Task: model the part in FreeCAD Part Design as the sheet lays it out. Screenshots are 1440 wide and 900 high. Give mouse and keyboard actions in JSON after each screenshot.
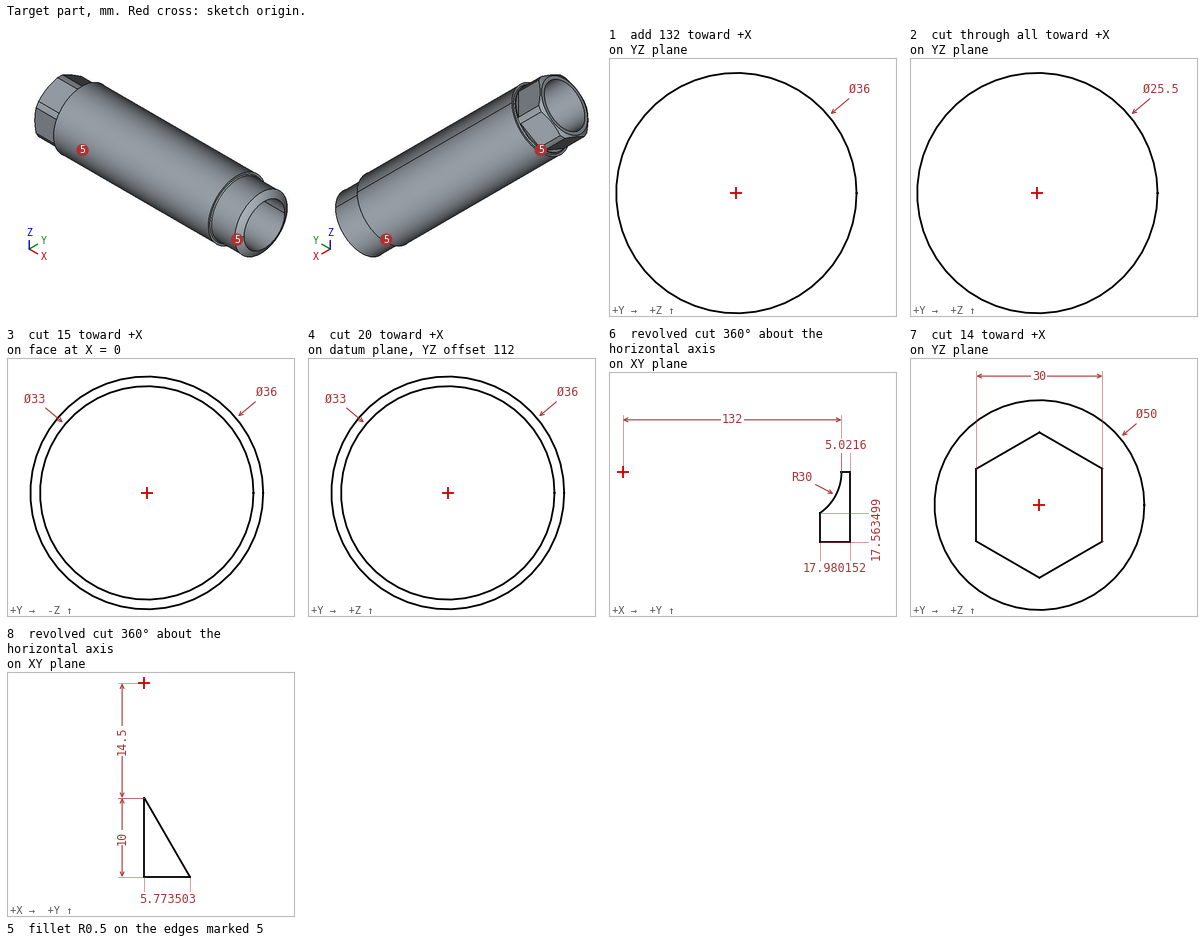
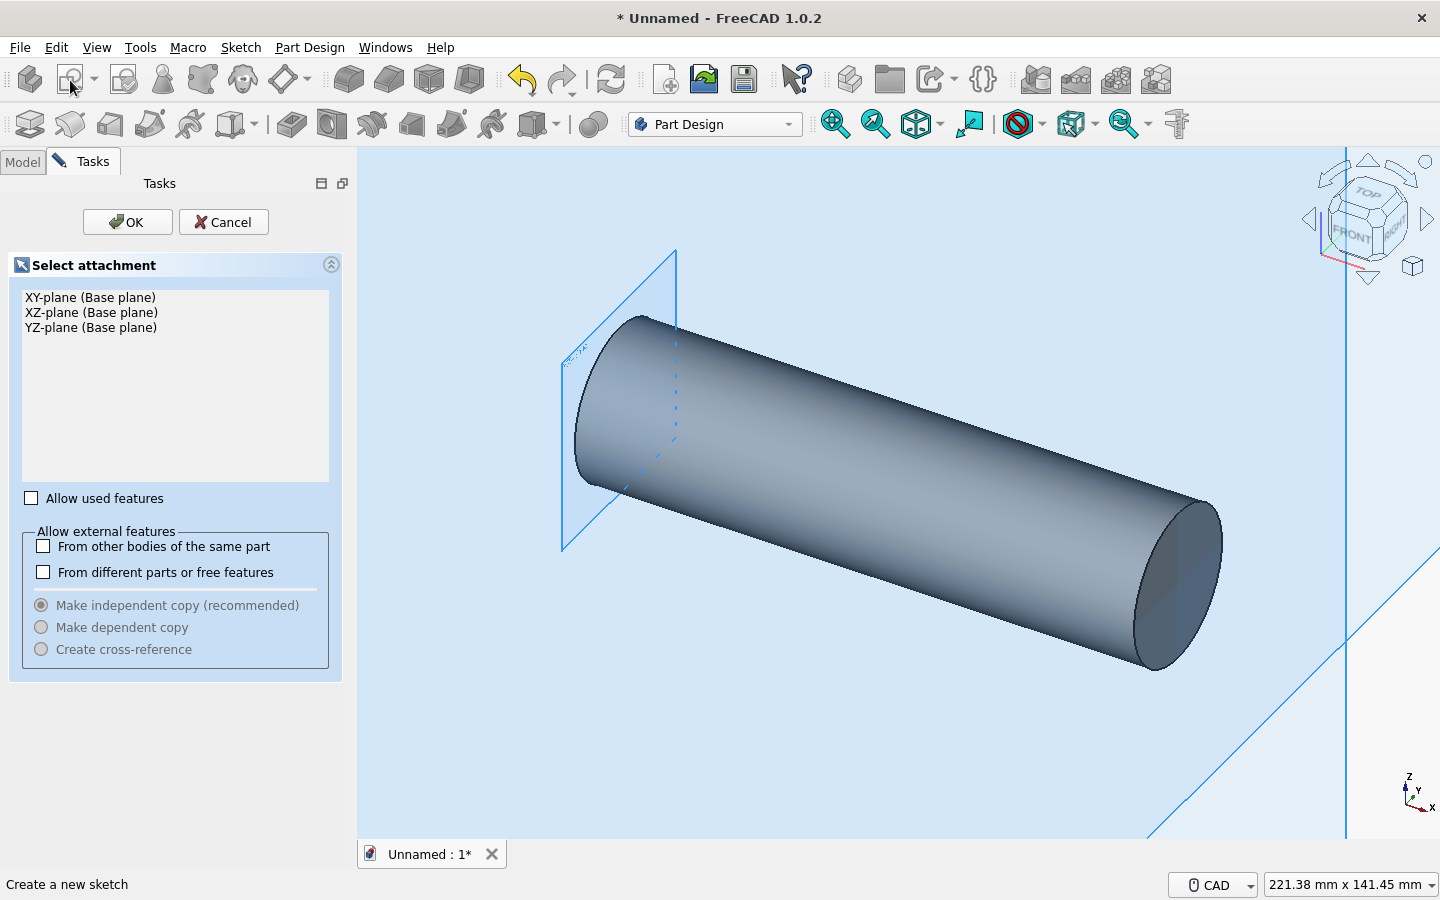
{"action": "left_click", "coordinate": [82, 328]}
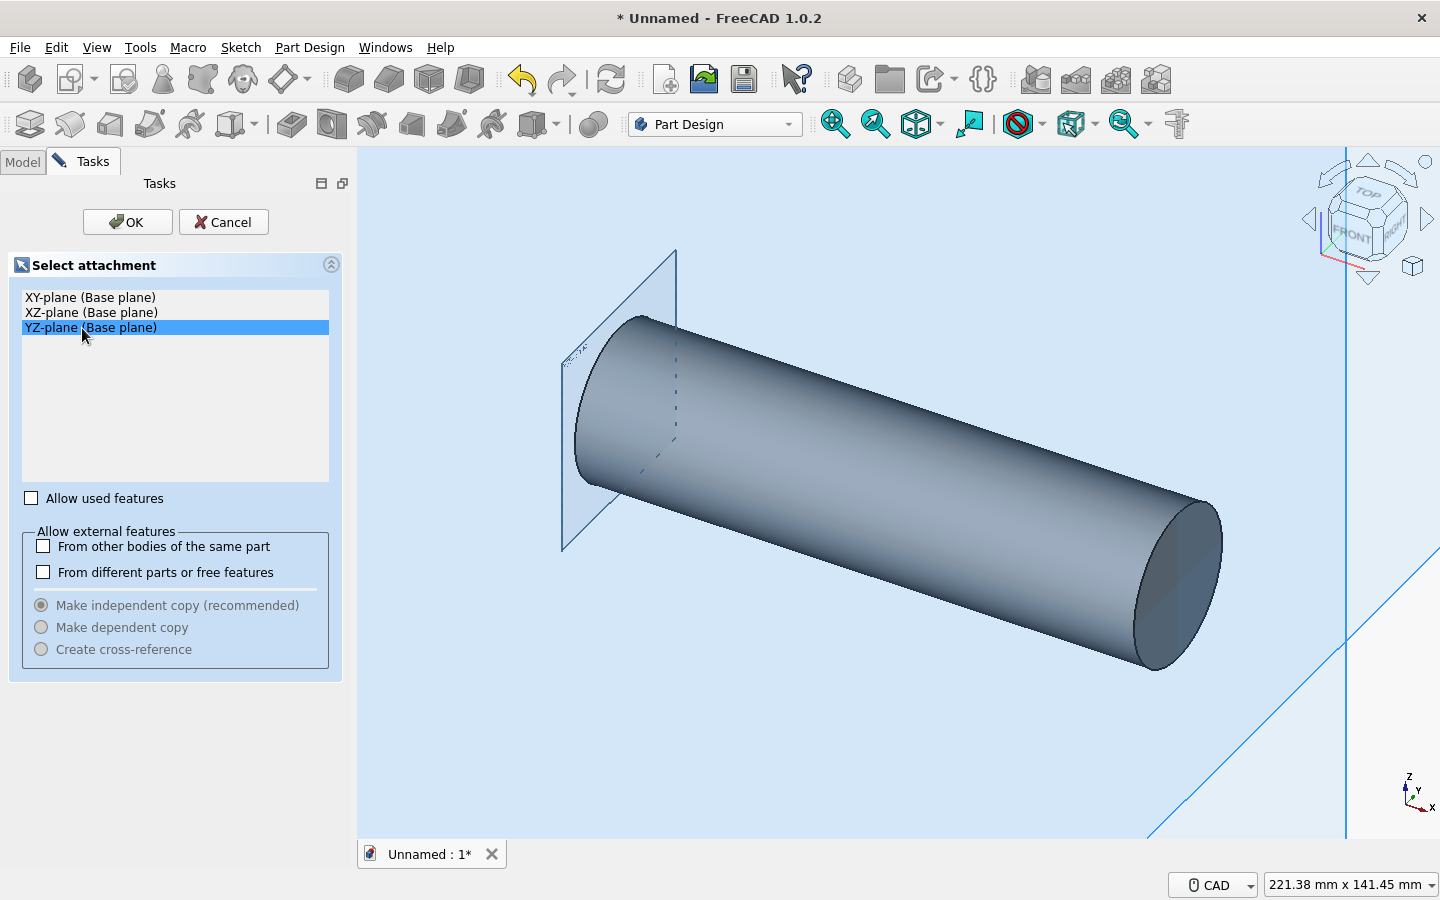
{"action": "left_click", "coordinate": [128, 222]}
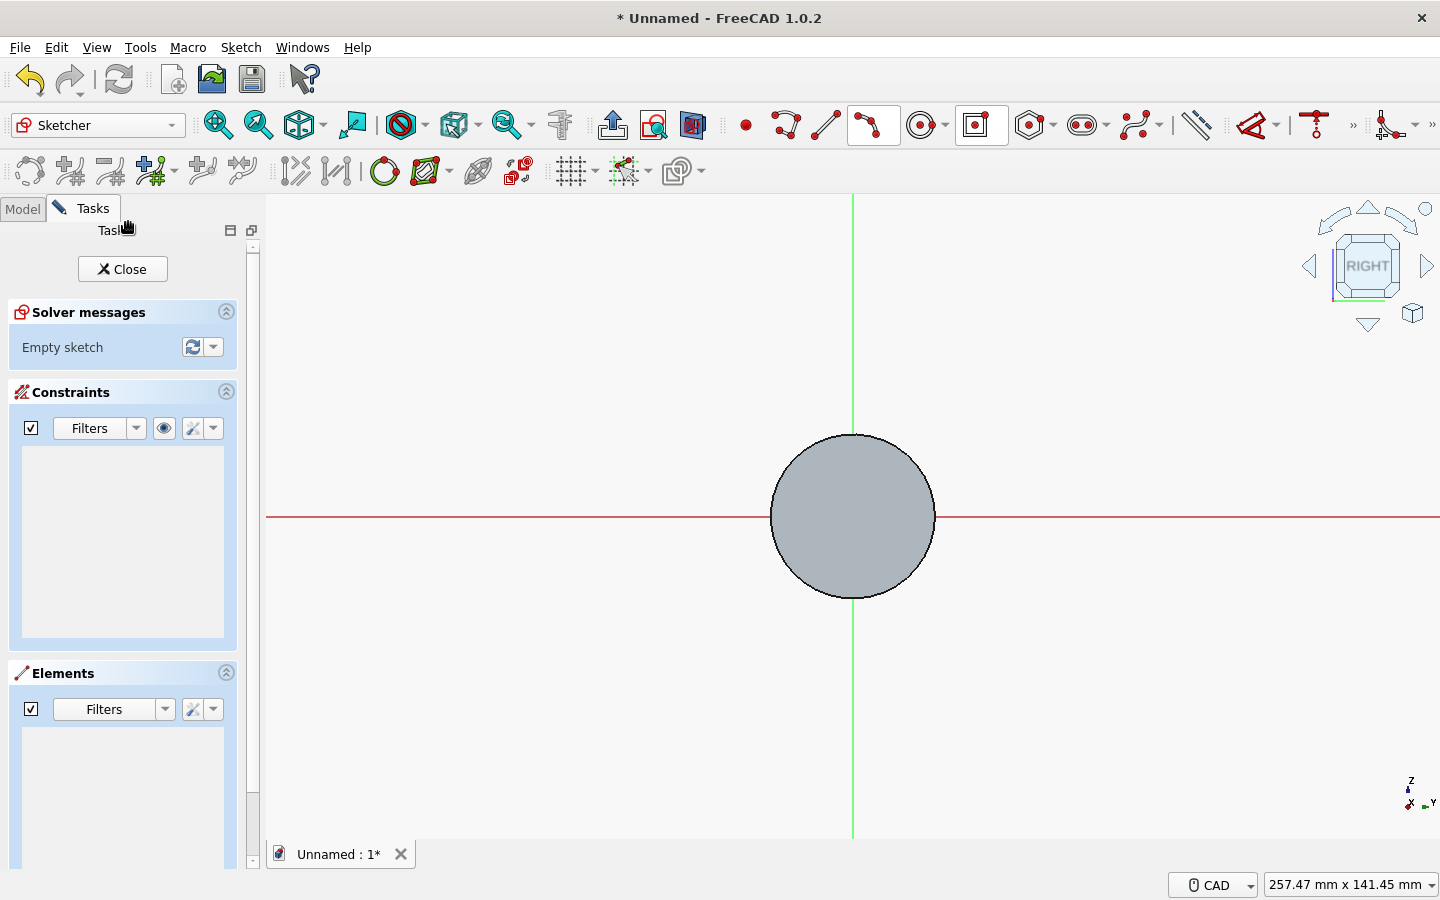
{"action": "key", "text": "q s"}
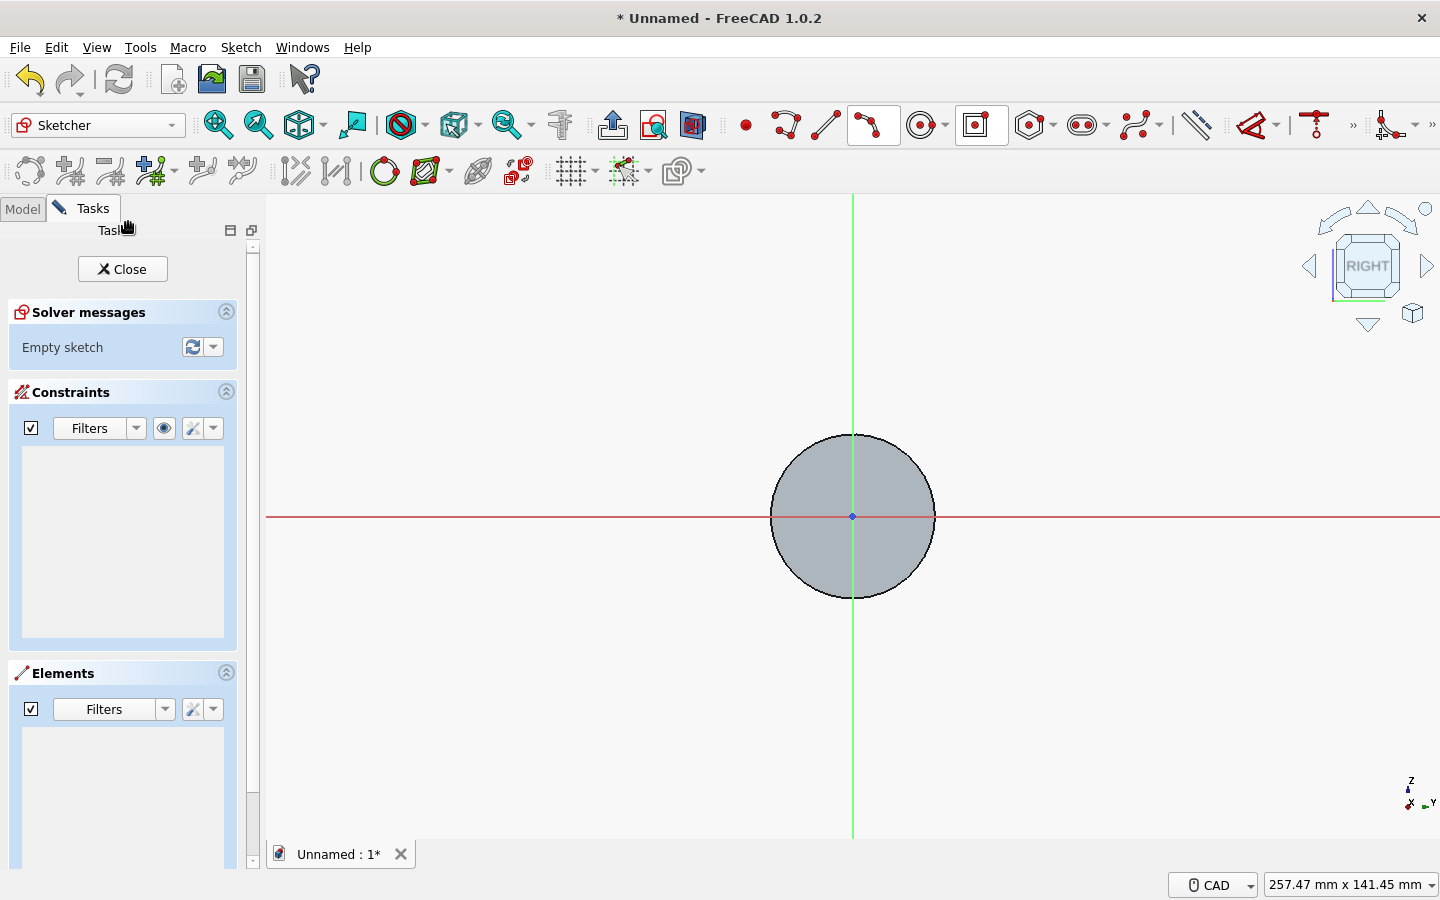
{"action": "scroll", "coordinate": [882, 516], "scroll_direction": "up", "scroll_amount": 6}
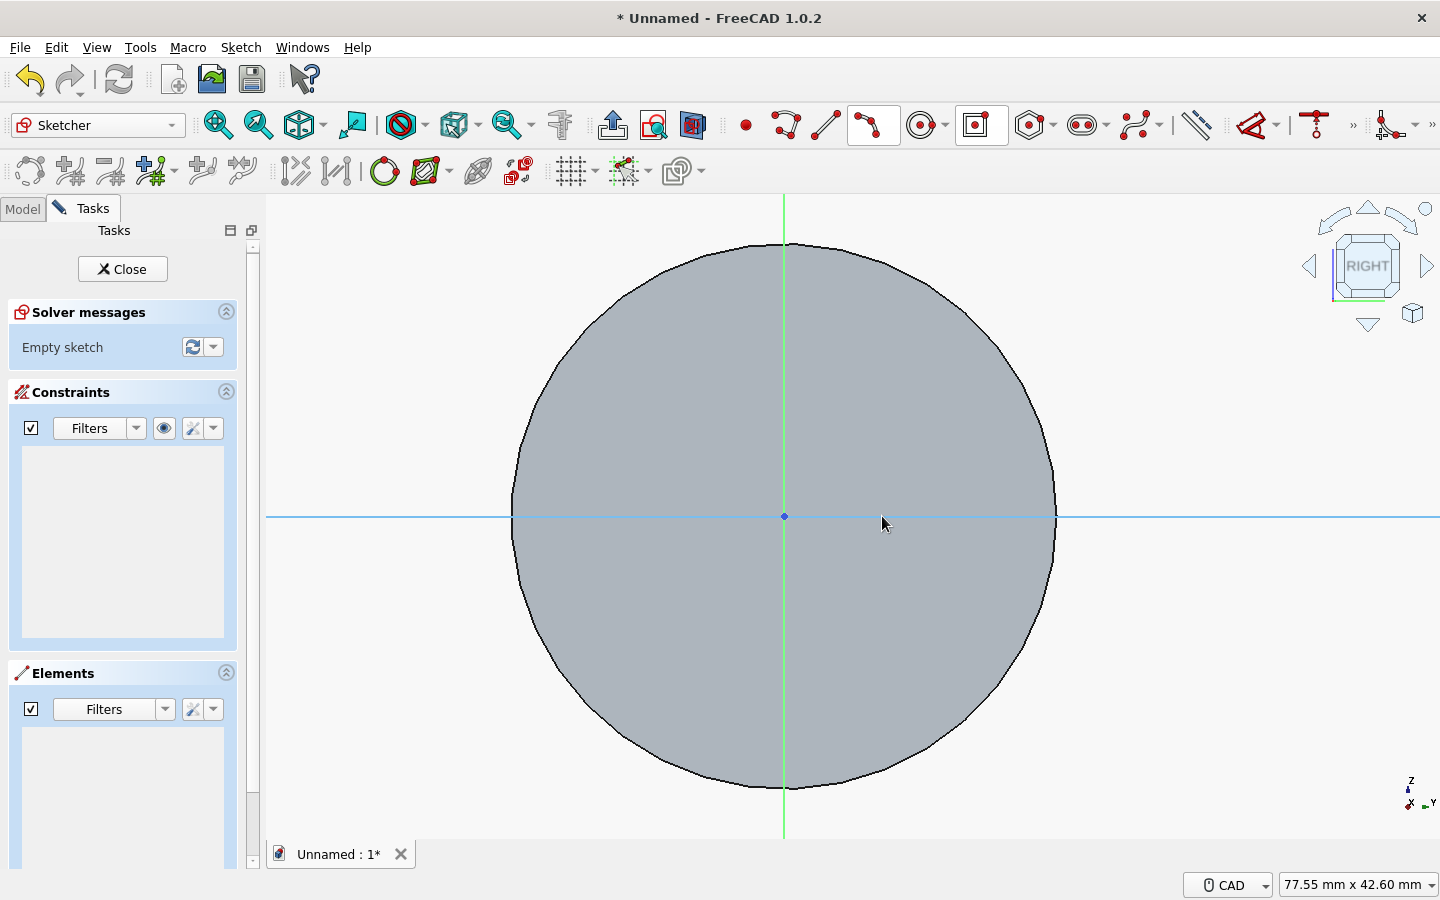
{"action": "left_click", "coordinate": [922, 126]}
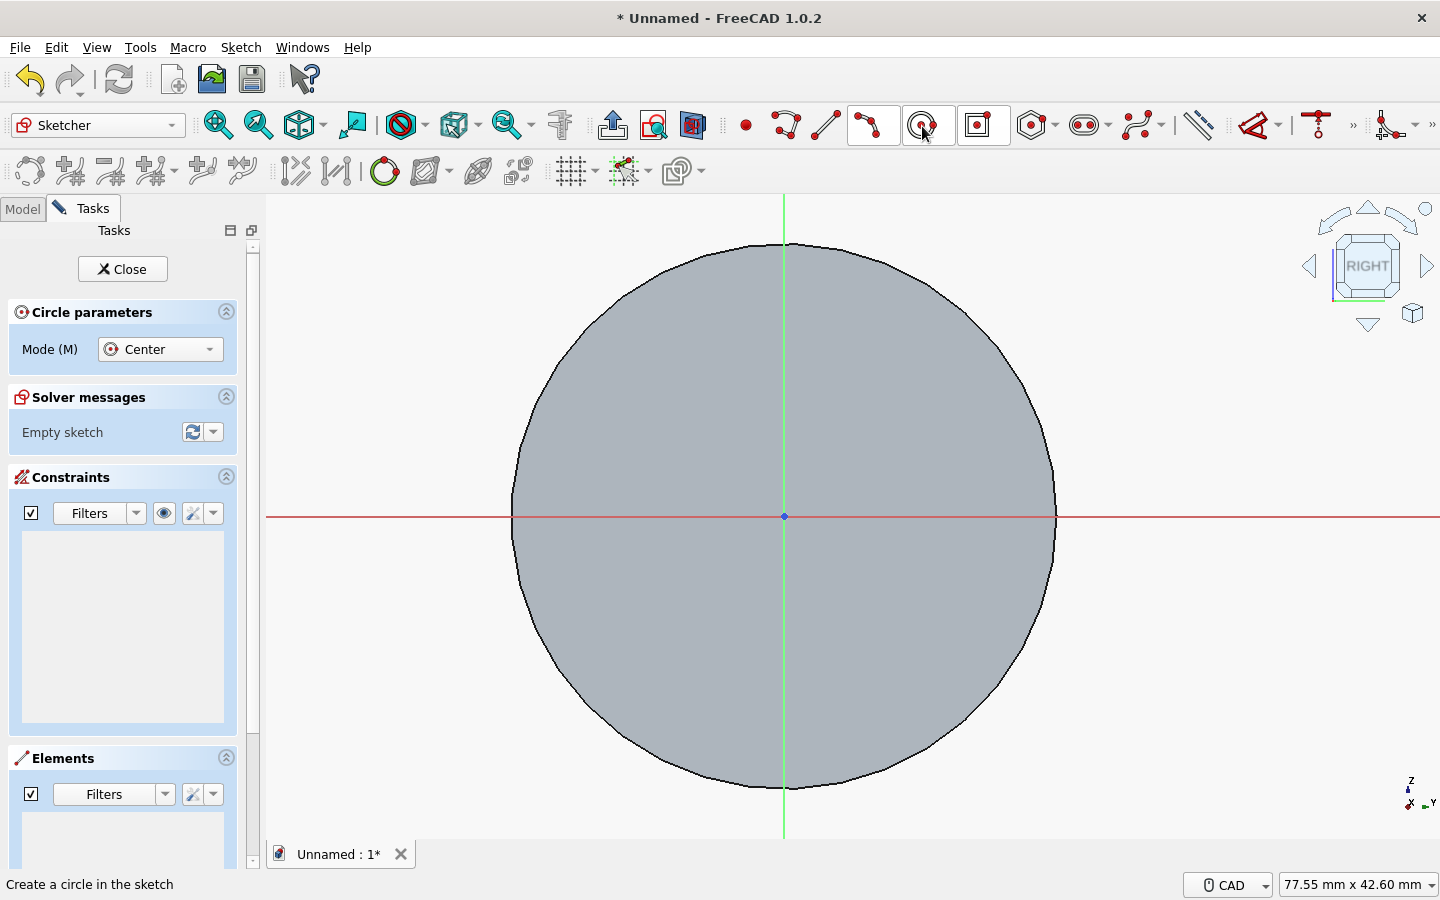
{"action": "left_click", "coordinate": [784, 516]}
{"action": "mouse_move", "coordinate": [920, 380]}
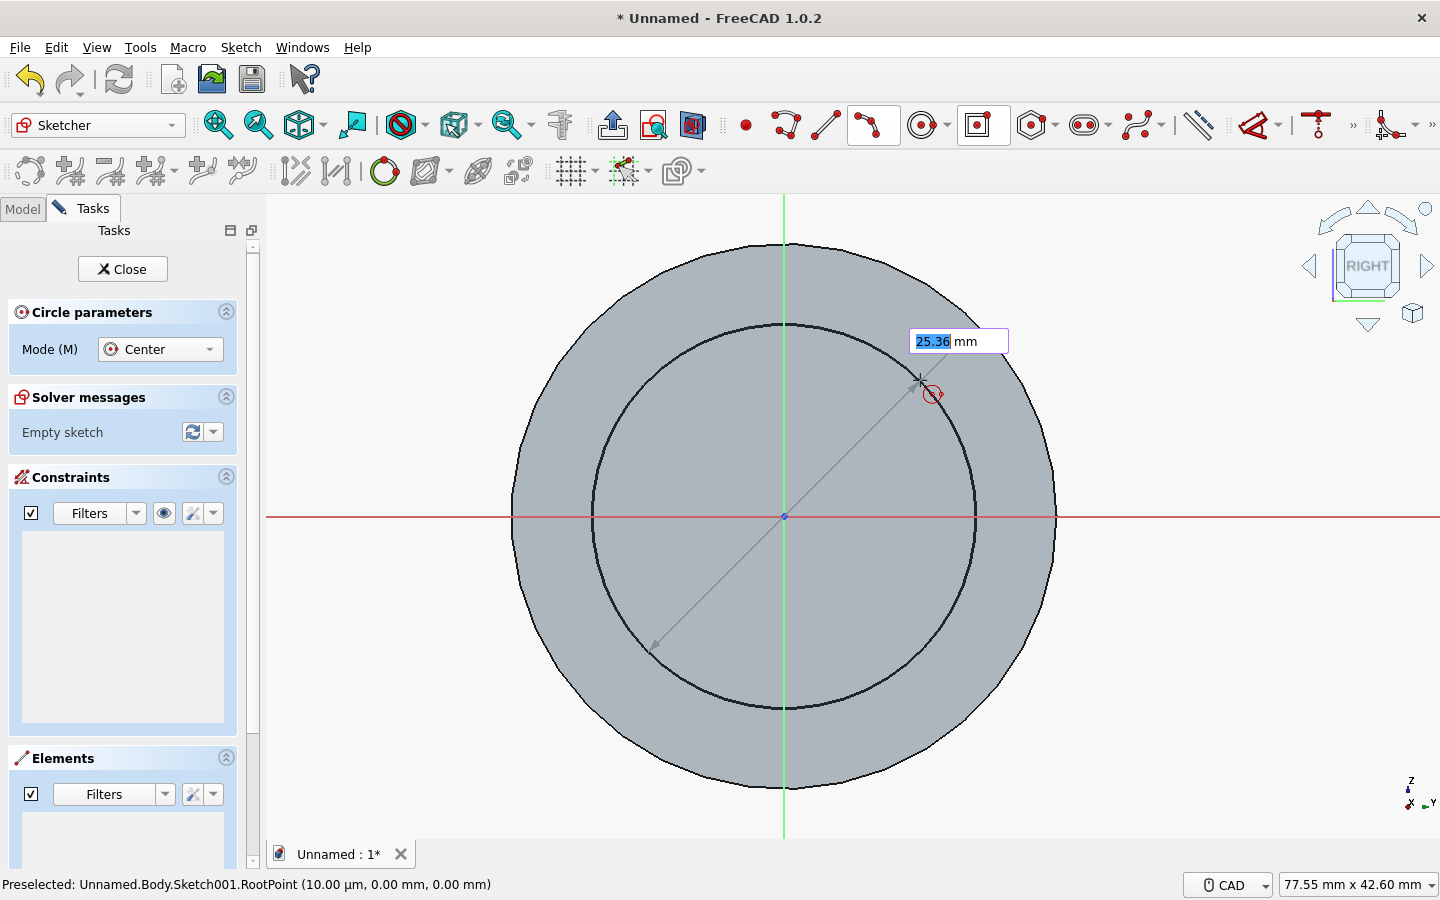
{"action": "type", "text": "25.5"}
{"action": "key", "text": "Return"}
{"action": "key", "text": "Escape"}